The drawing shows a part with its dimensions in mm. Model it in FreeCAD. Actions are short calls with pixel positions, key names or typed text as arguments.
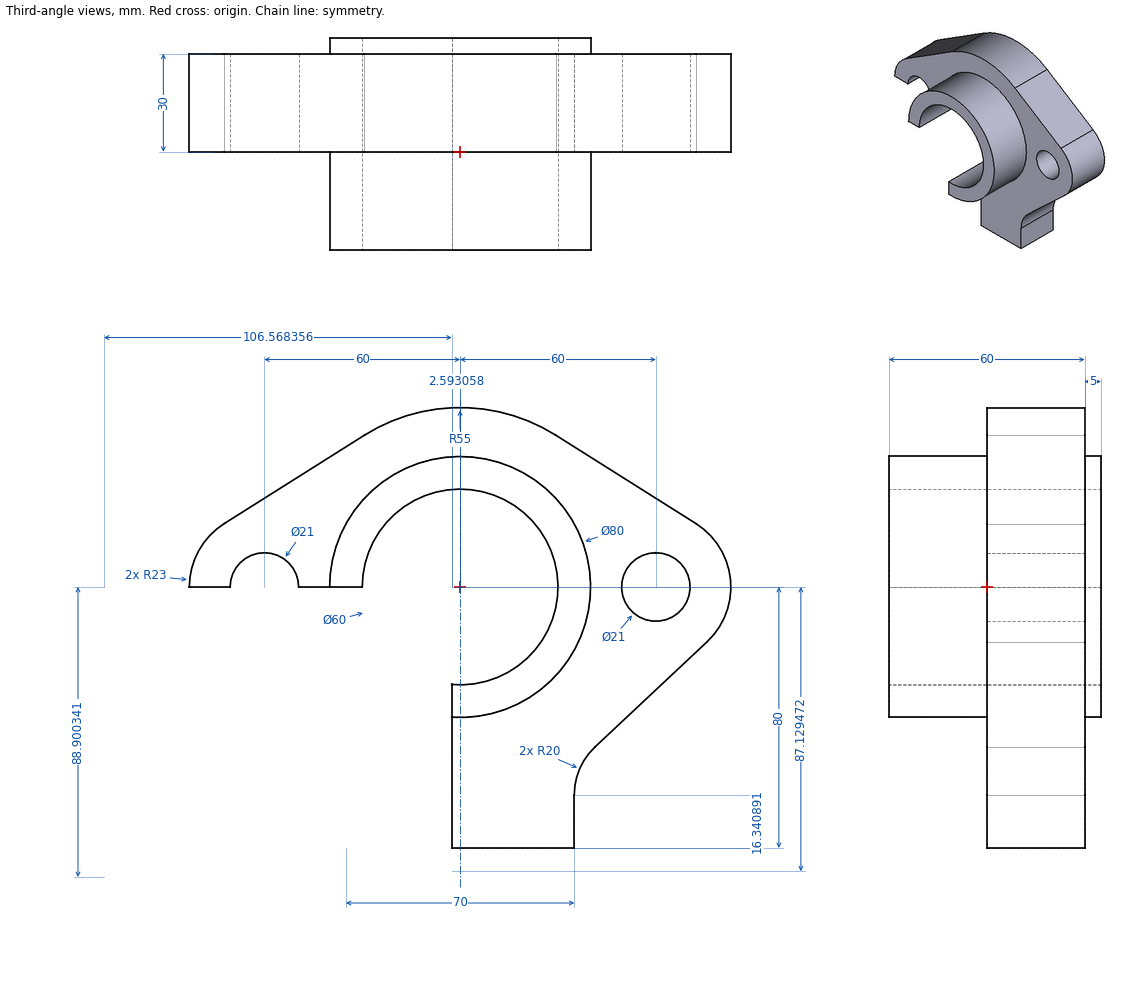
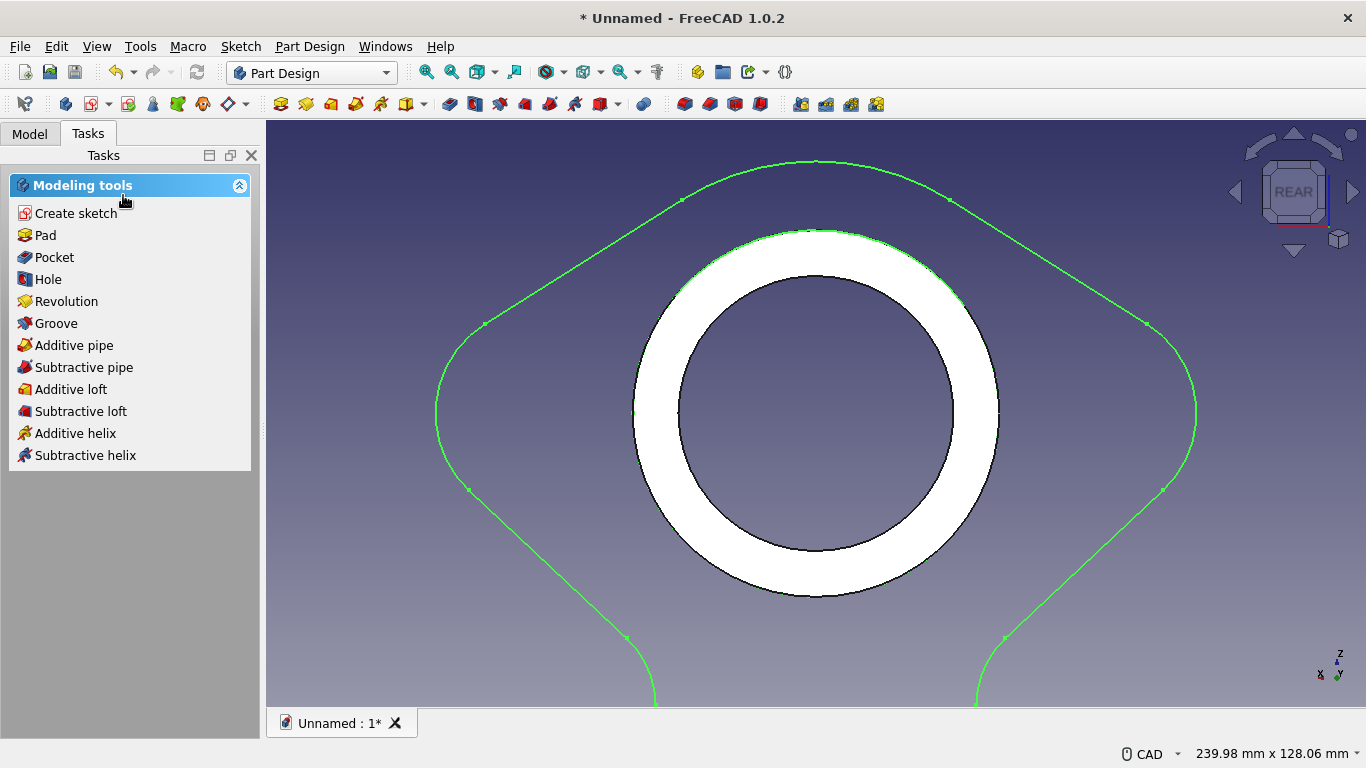
click(281, 104)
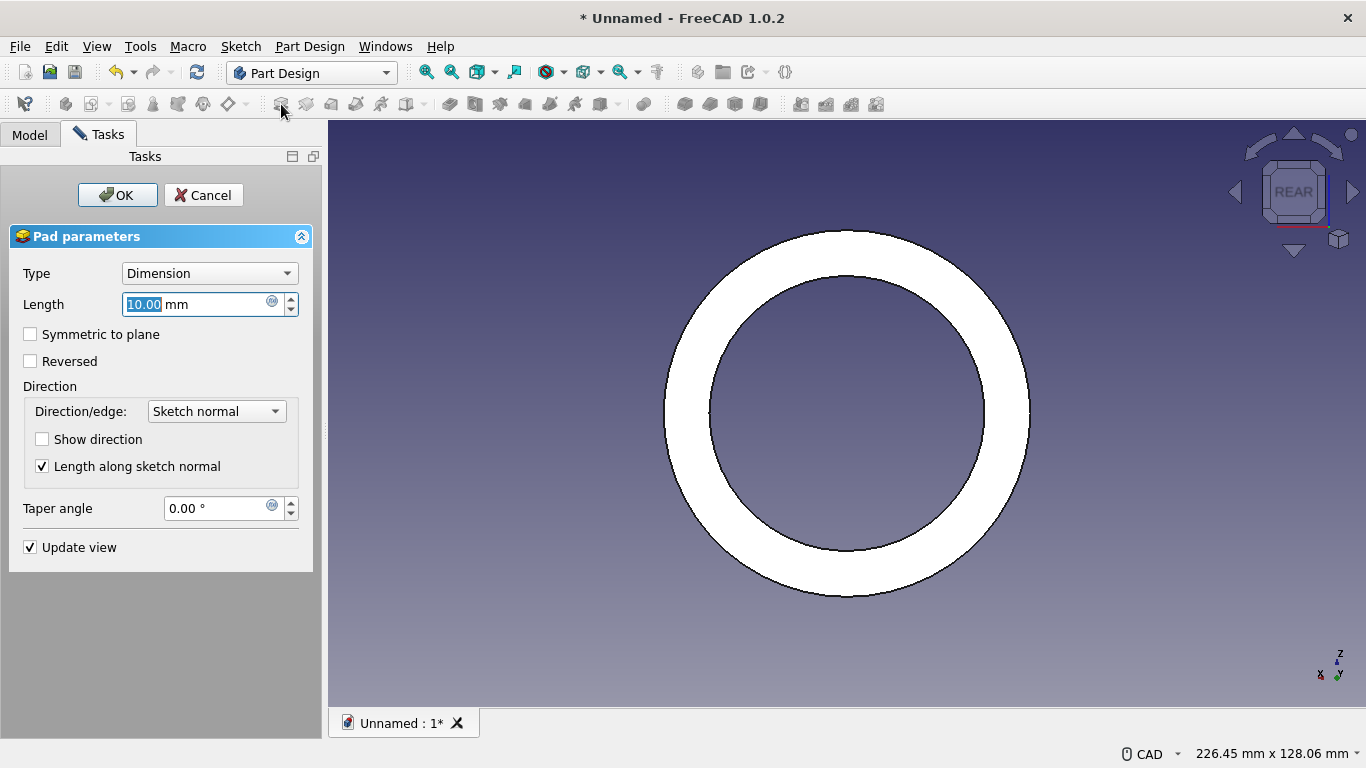
text(30)
key(Tab)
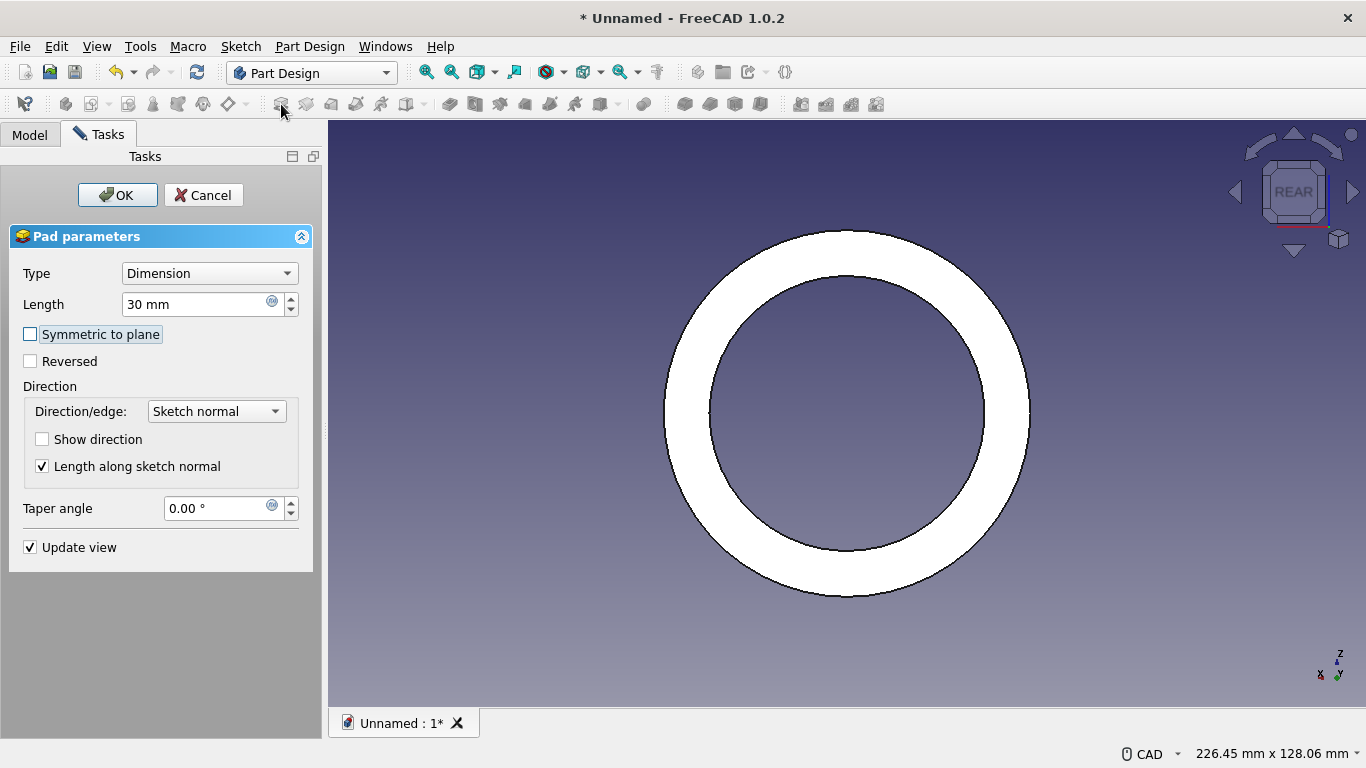
click(31, 361)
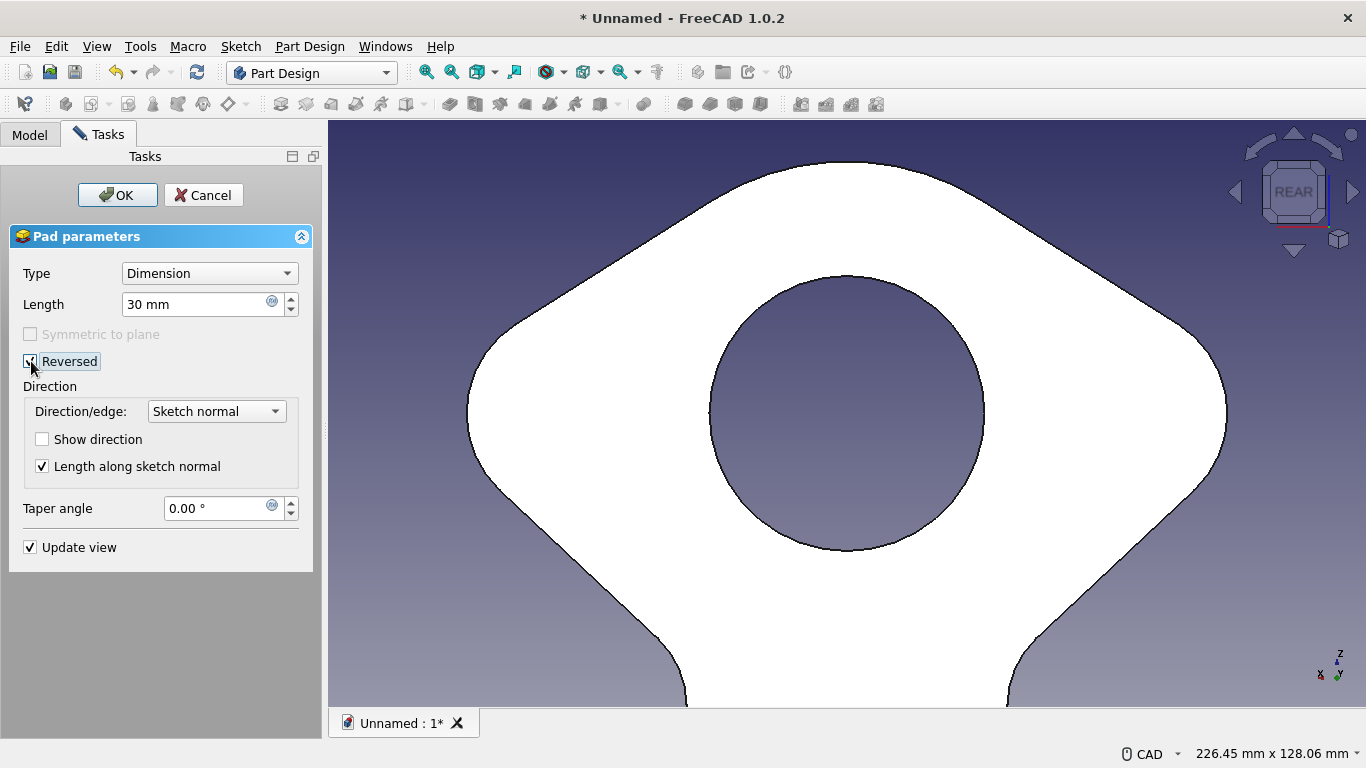
click(118, 195)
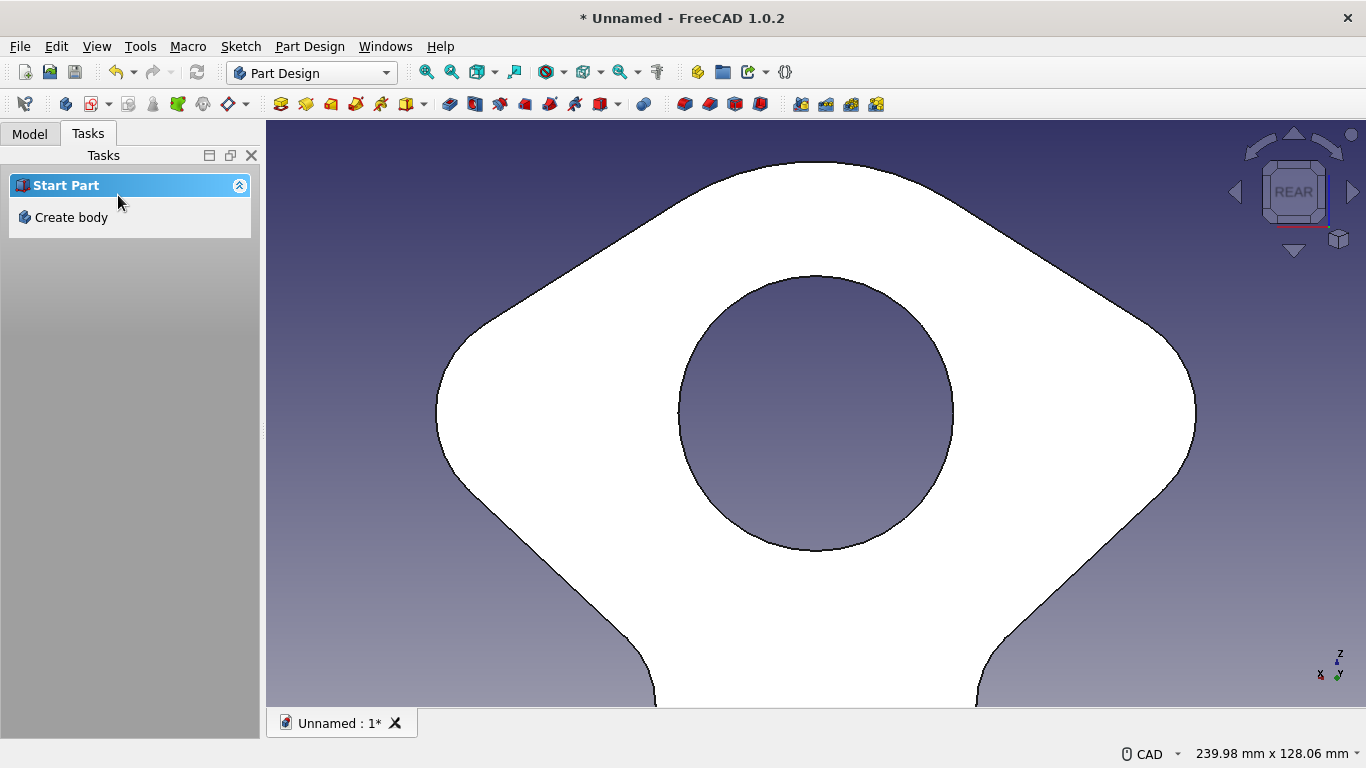
click(427, 72)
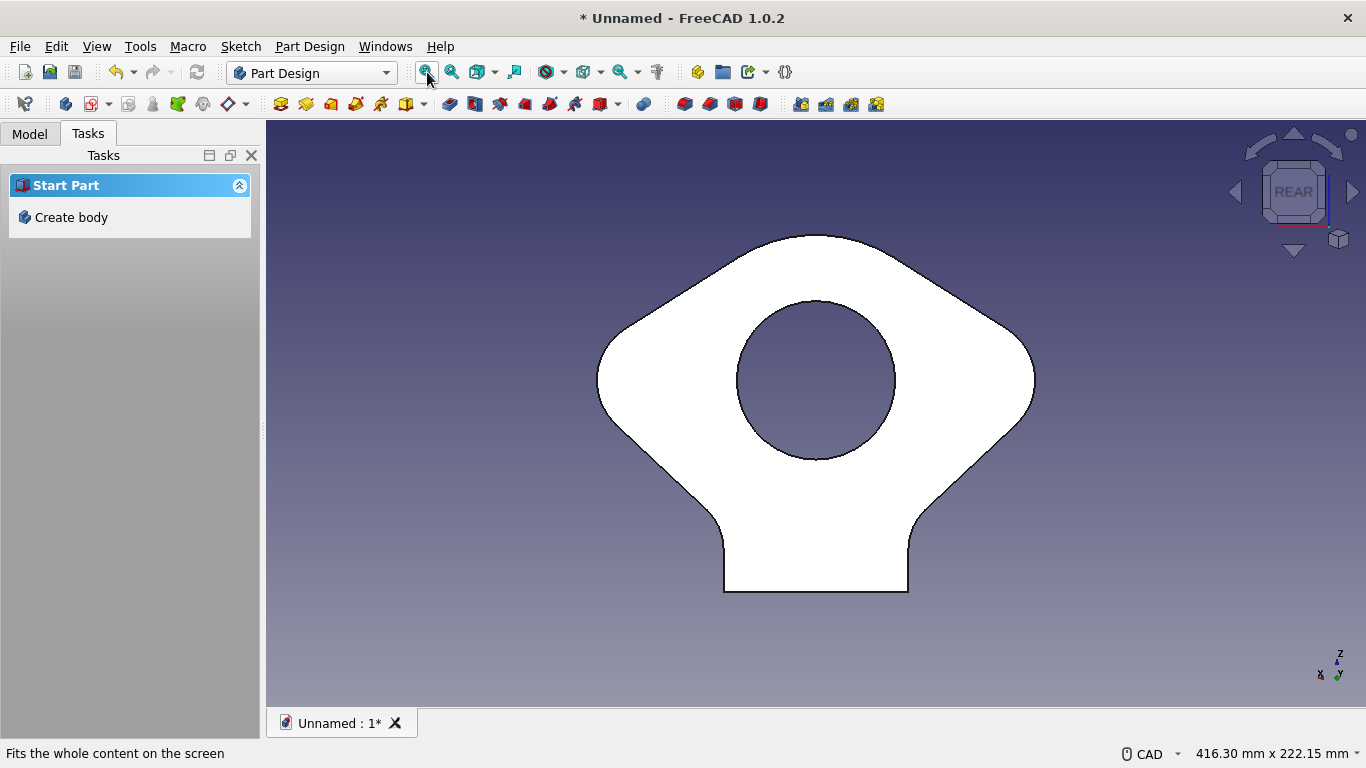
click(816, 514)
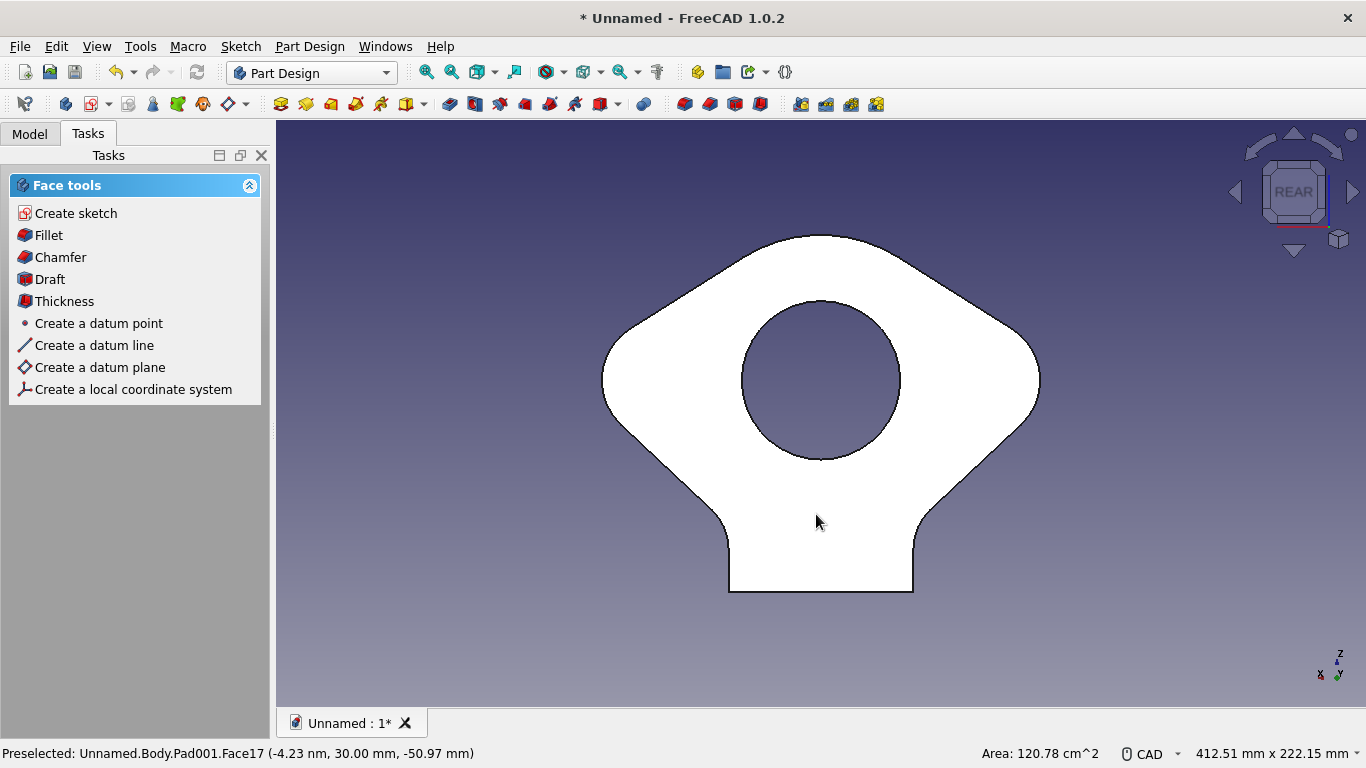
click(90, 104)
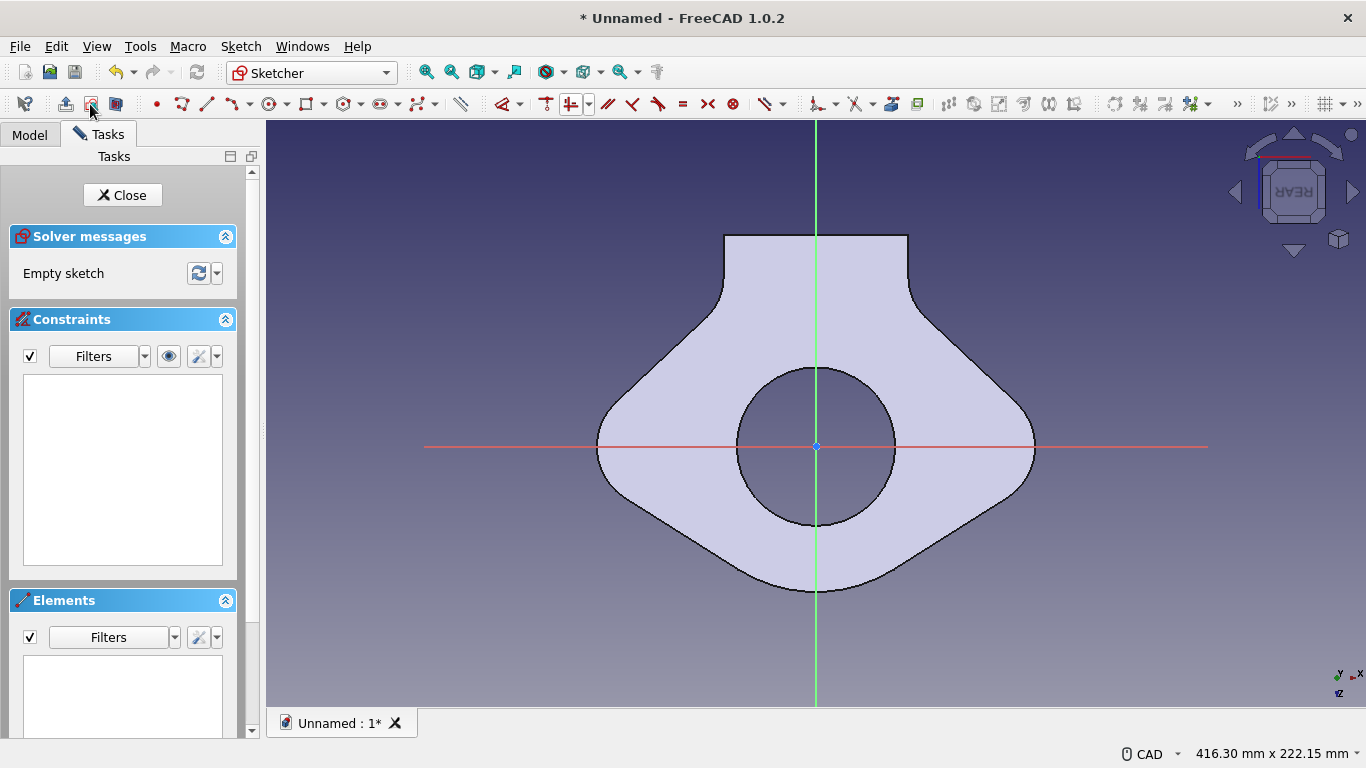
scroll(899, 487, up, 3)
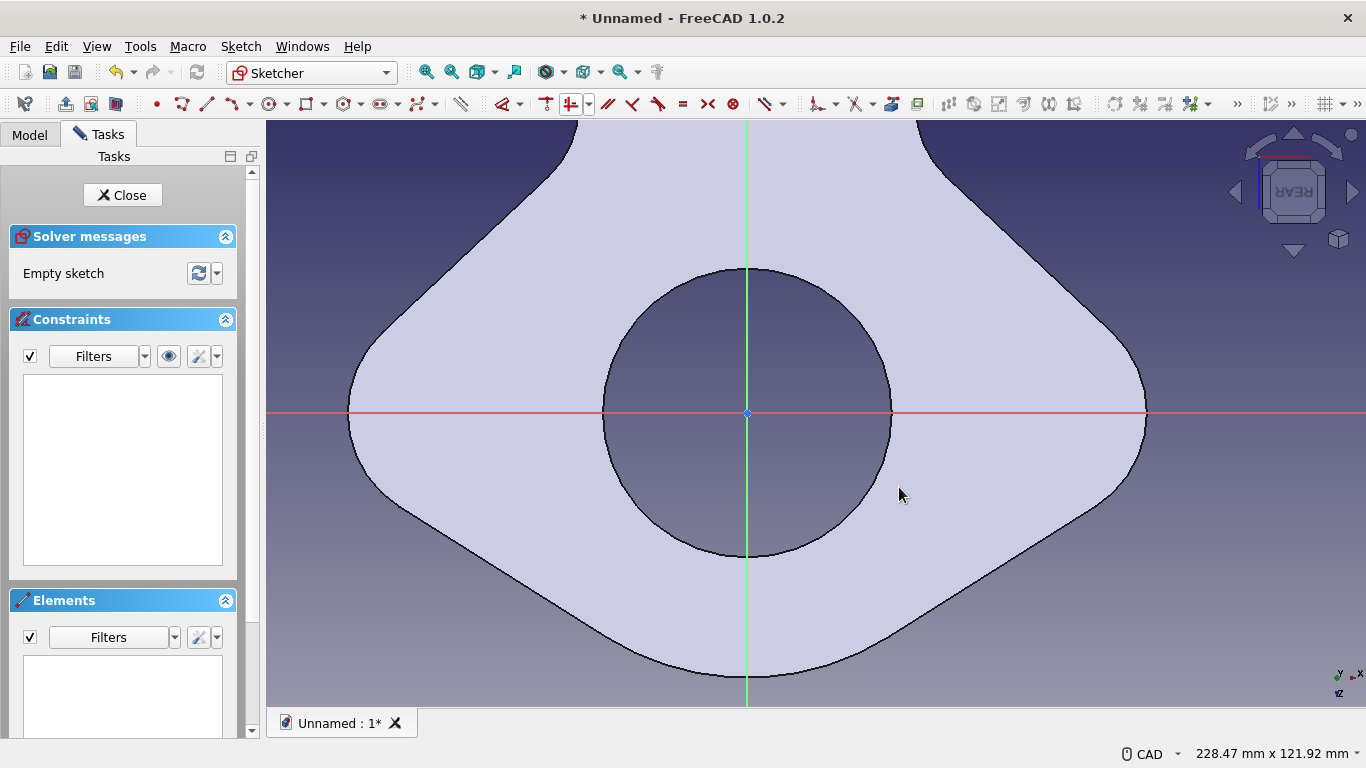
click(268, 104)